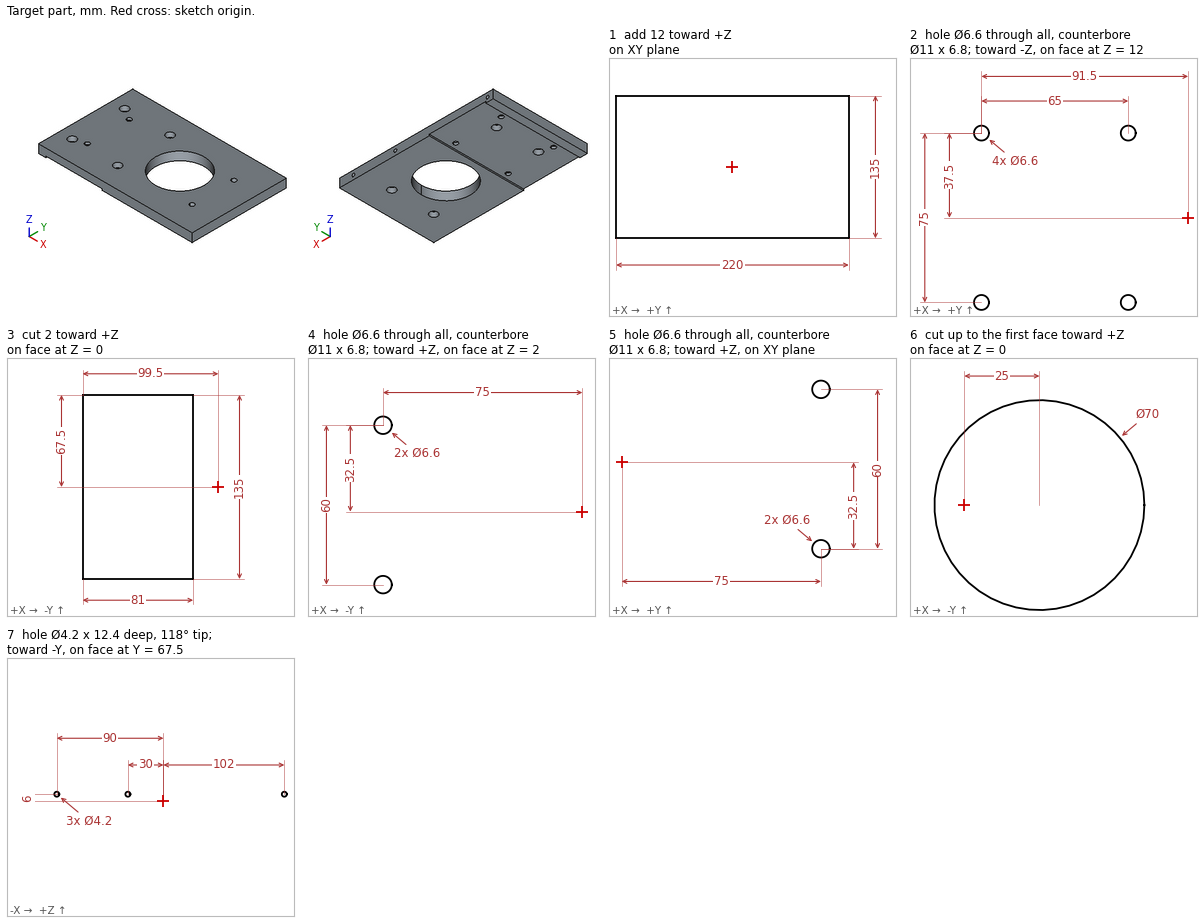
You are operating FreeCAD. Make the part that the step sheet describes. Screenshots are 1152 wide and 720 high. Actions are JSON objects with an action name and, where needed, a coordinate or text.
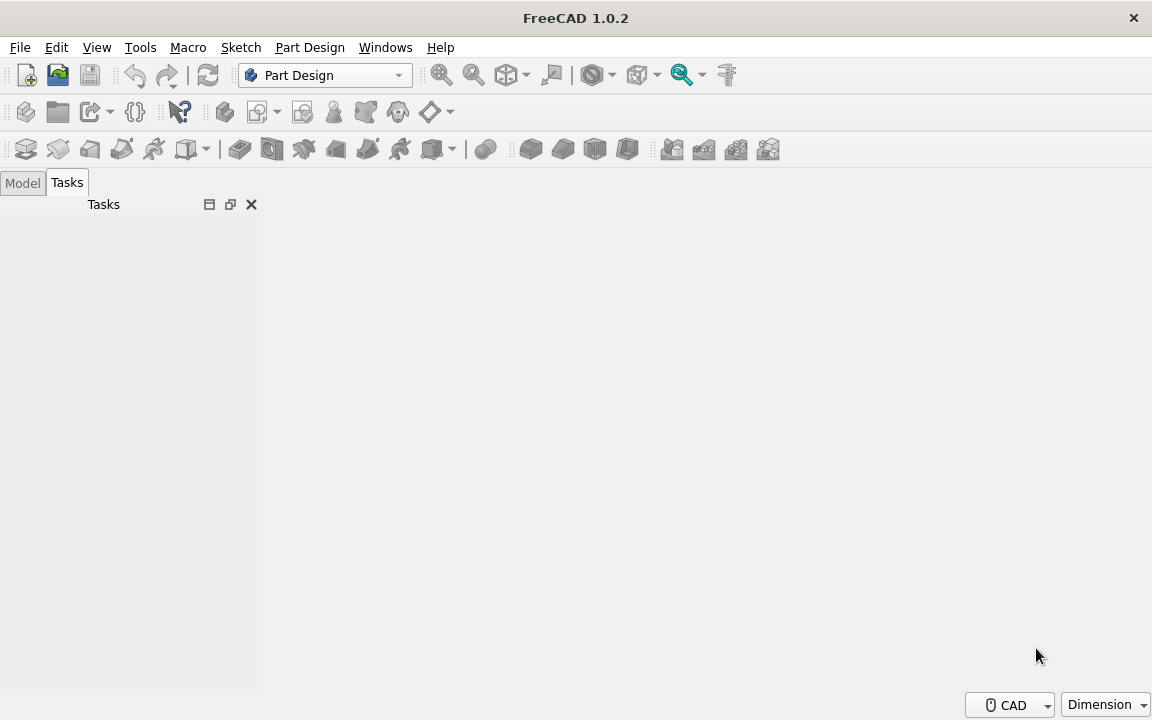
{"action": "key", "text": "ctrl+n"}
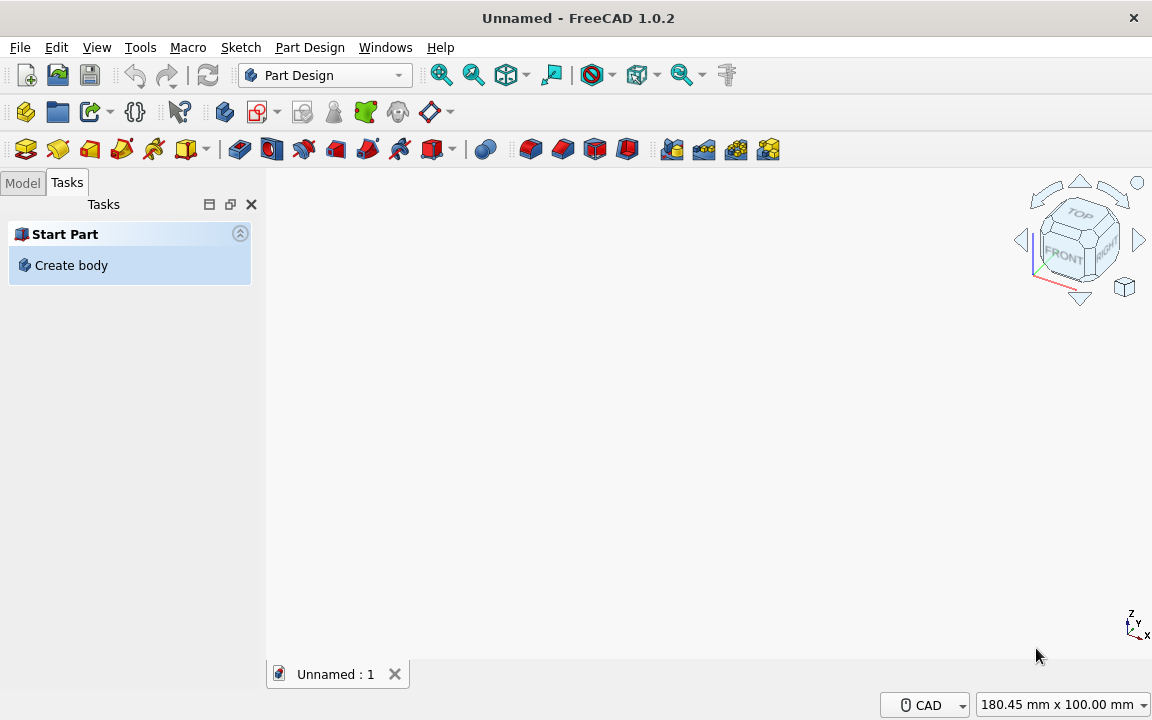
{"action": "left_click", "coordinate": [258, 112]}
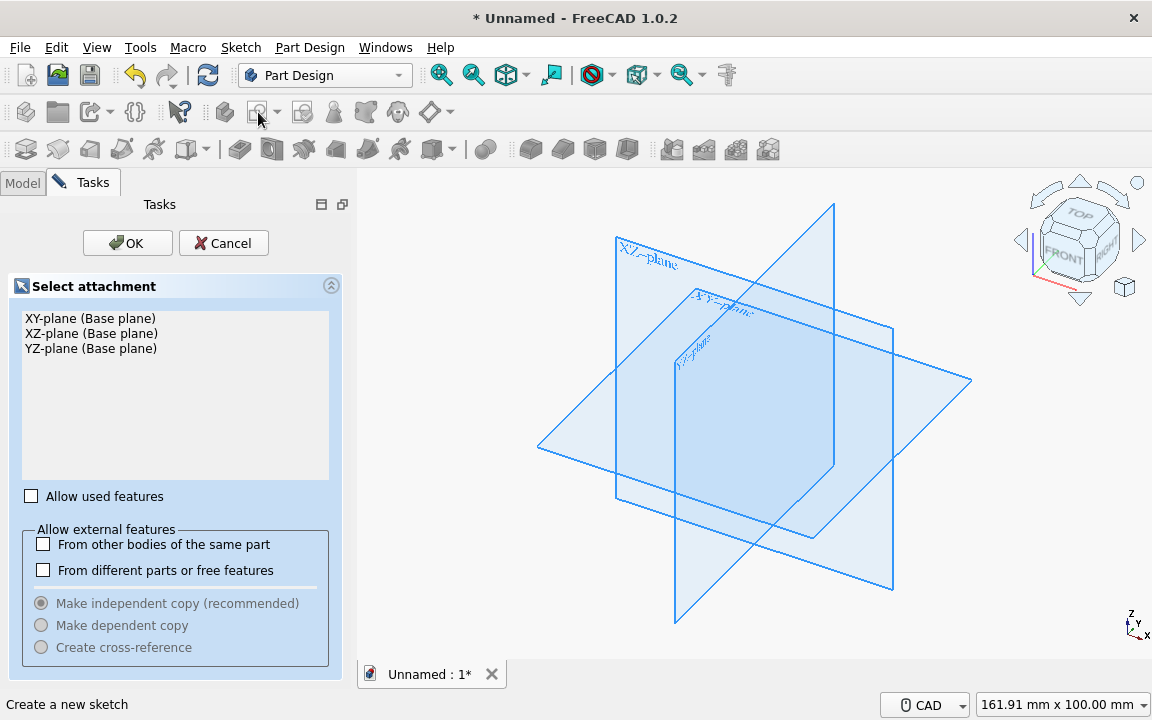
{"action": "left_click", "coordinate": [82, 318]}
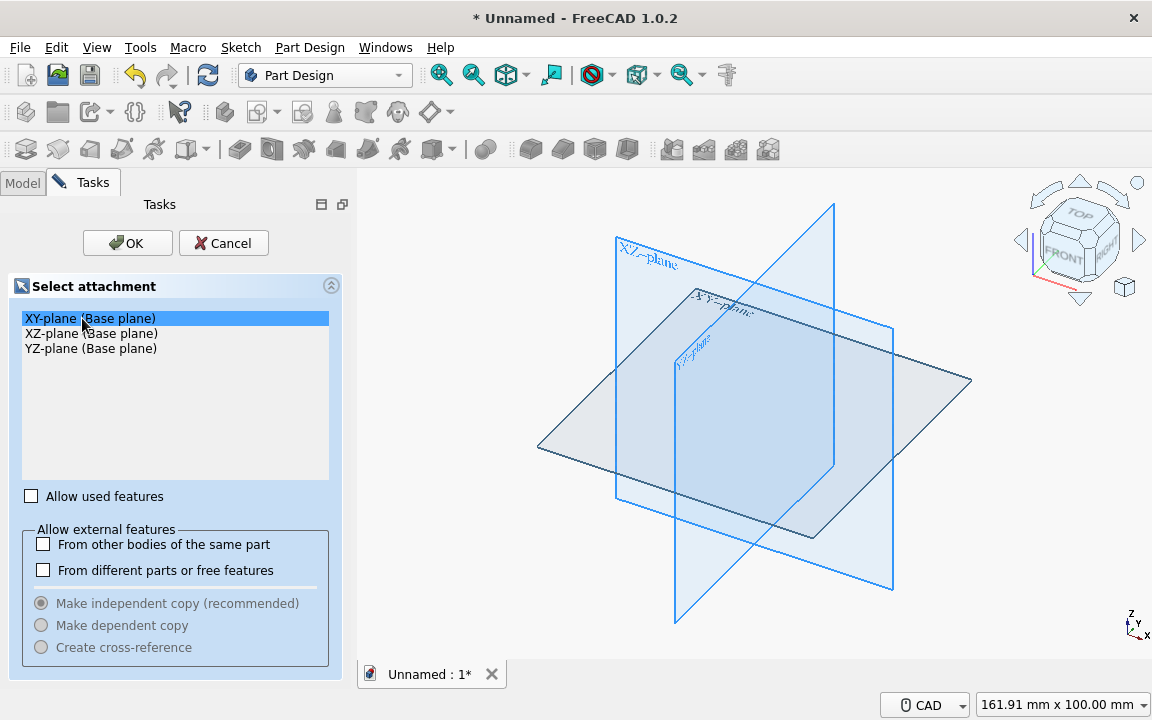
{"action": "left_click", "coordinate": [128, 243]}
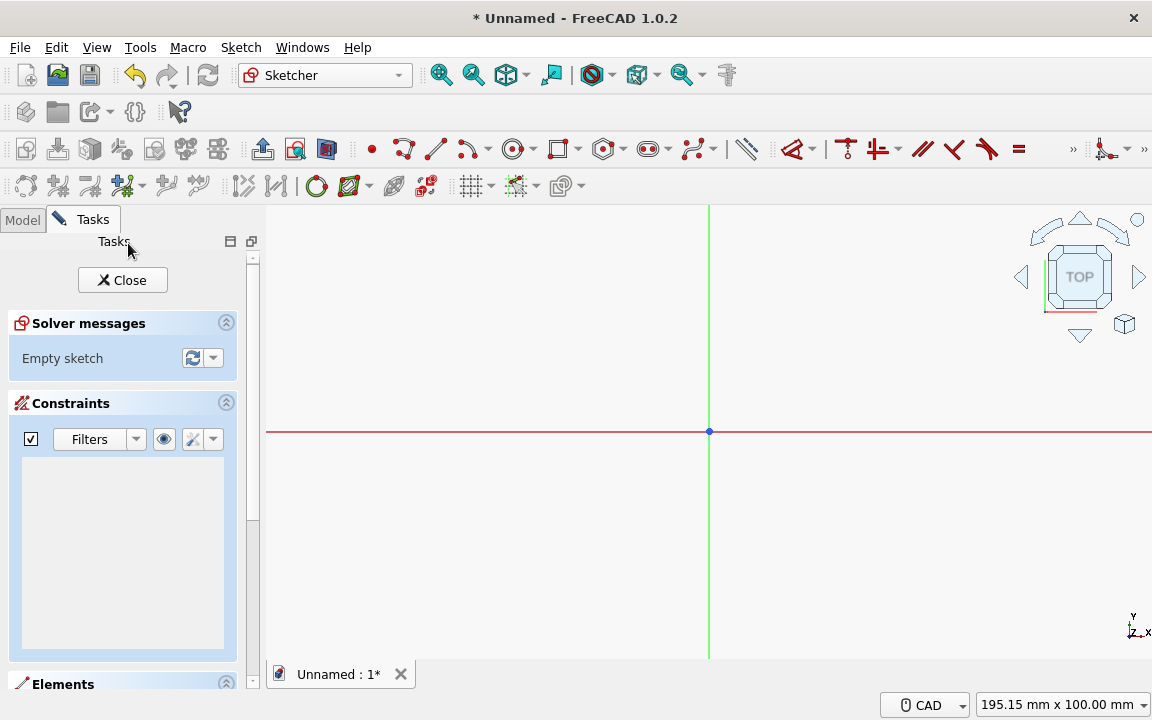
{"action": "scroll", "coordinate": [585, 432], "scroll_direction": "down", "scroll_amount": 4}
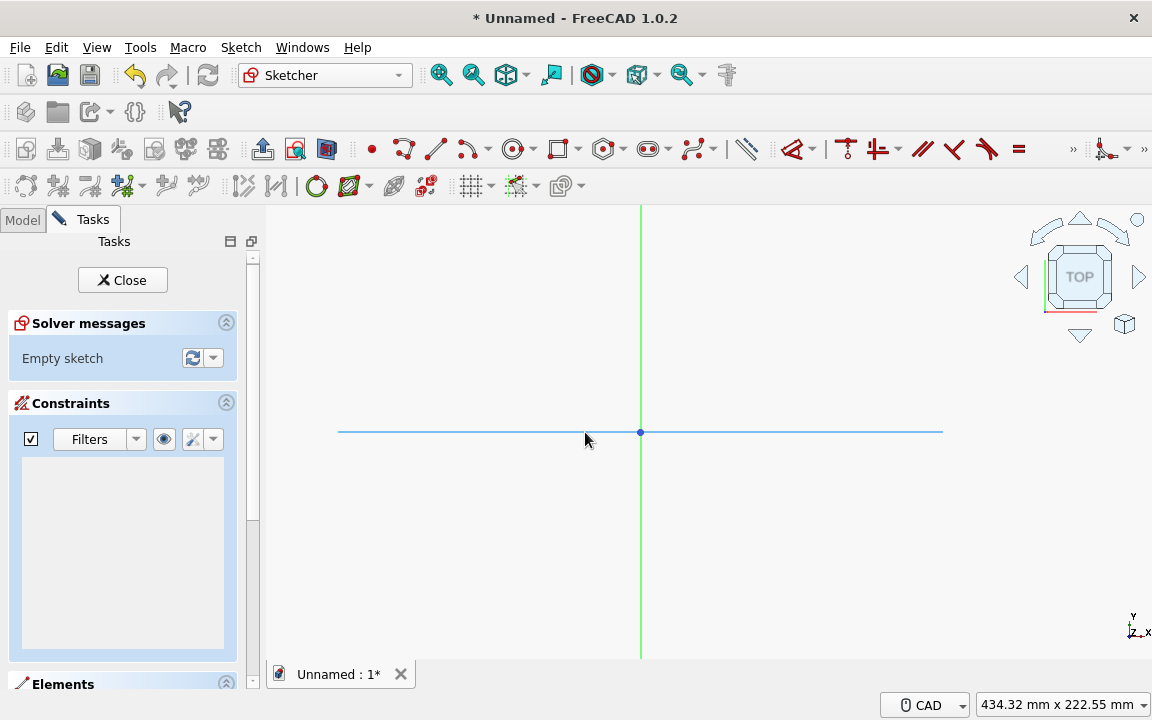
{"action": "left_click", "coordinate": [580, 150]}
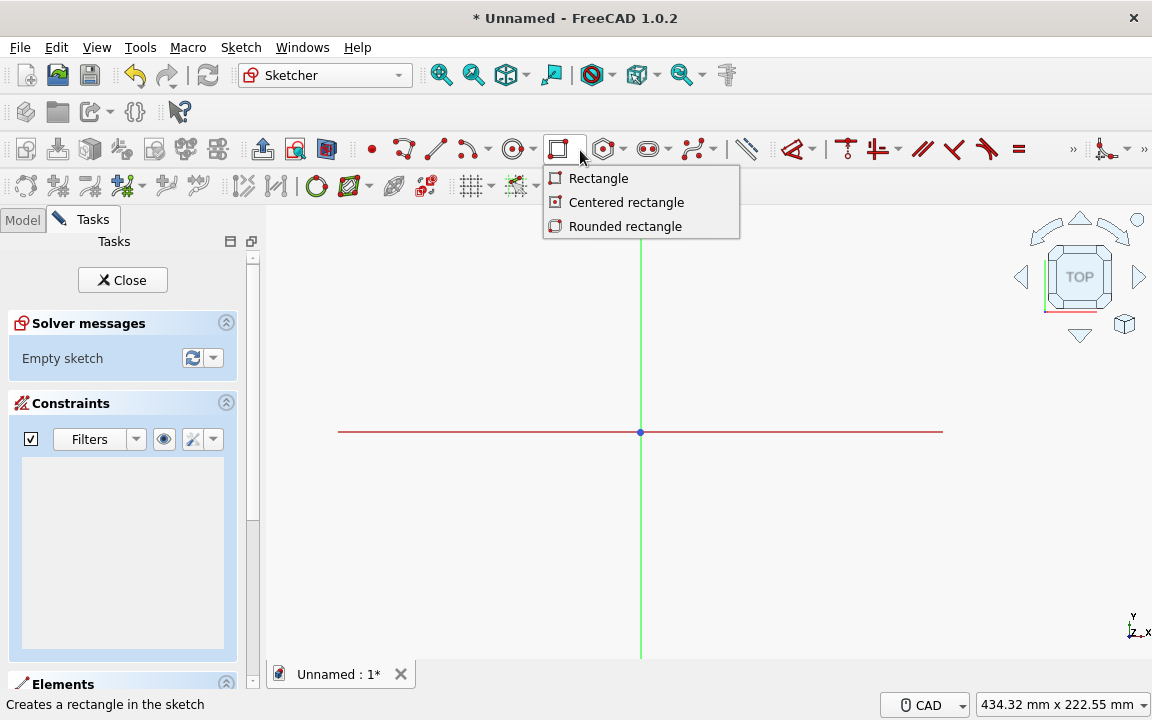
{"action": "left_click", "coordinate": [642, 202]}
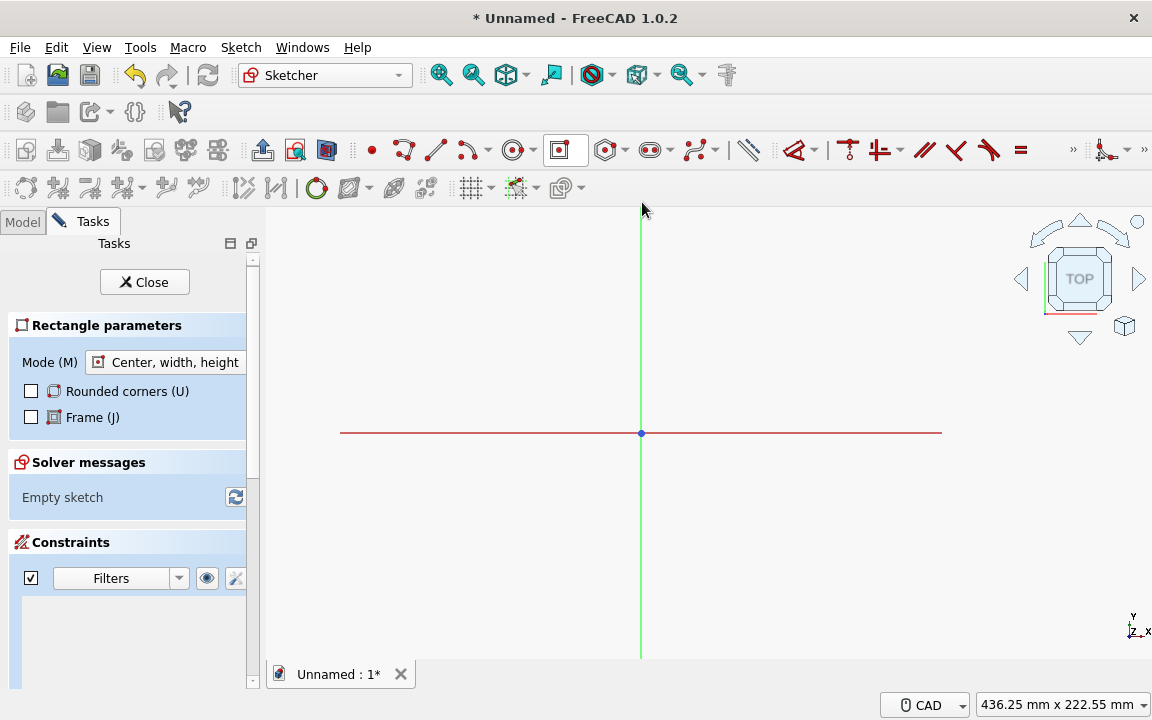
{"action": "left_click", "coordinate": [641, 433]}
{"action": "mouse_move", "coordinate": [865, 296]}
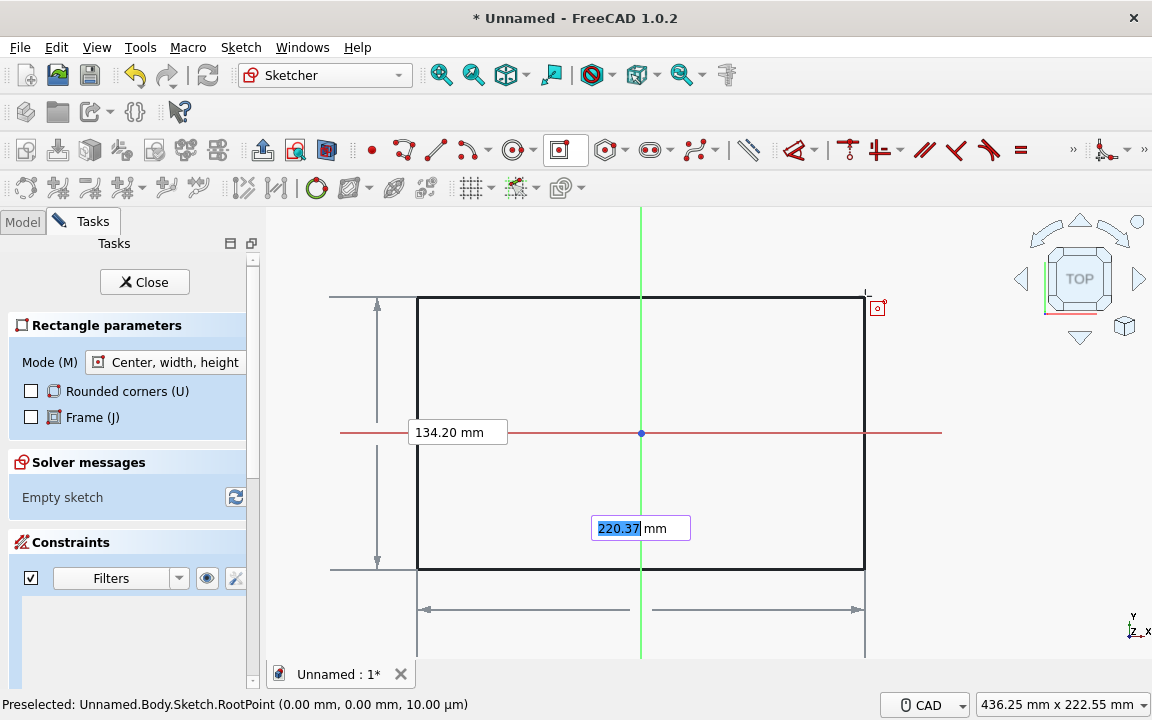
{"action": "type", "text": "220"}
{"action": "key", "text": "Tab"}
{"action": "type", "text": "135"}
{"action": "key", "text": "Return"}
{"action": "key", "text": "Escape"}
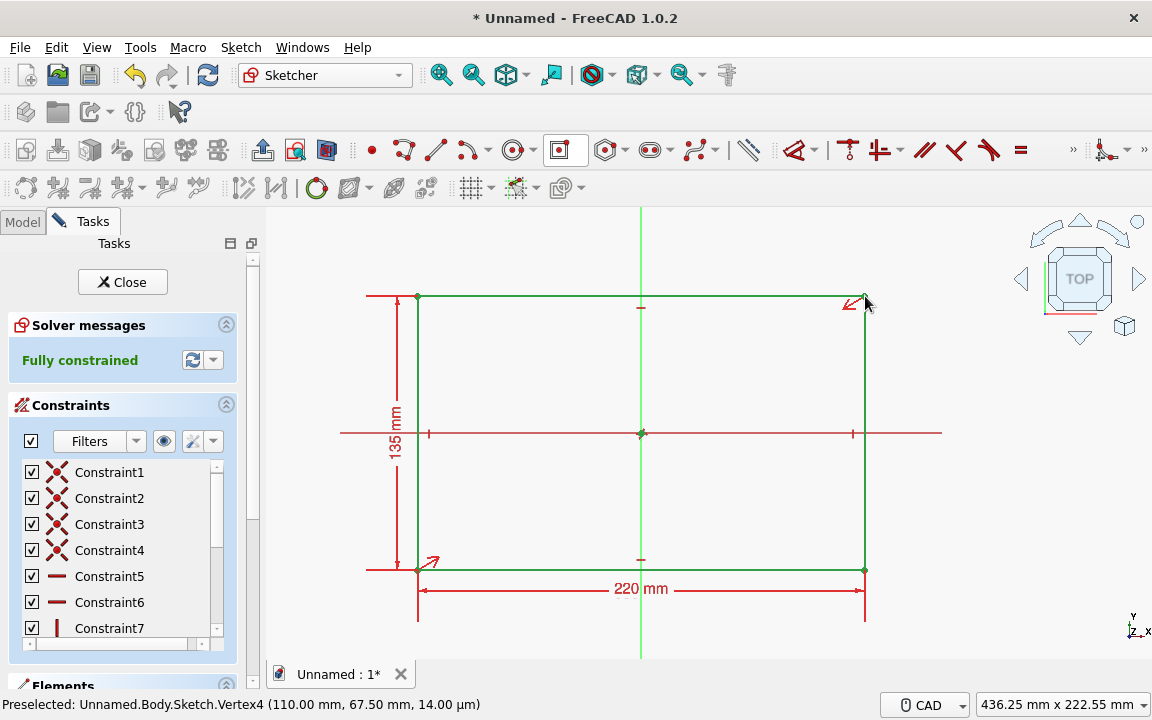
{"action": "left_click", "coordinate": [123, 282]}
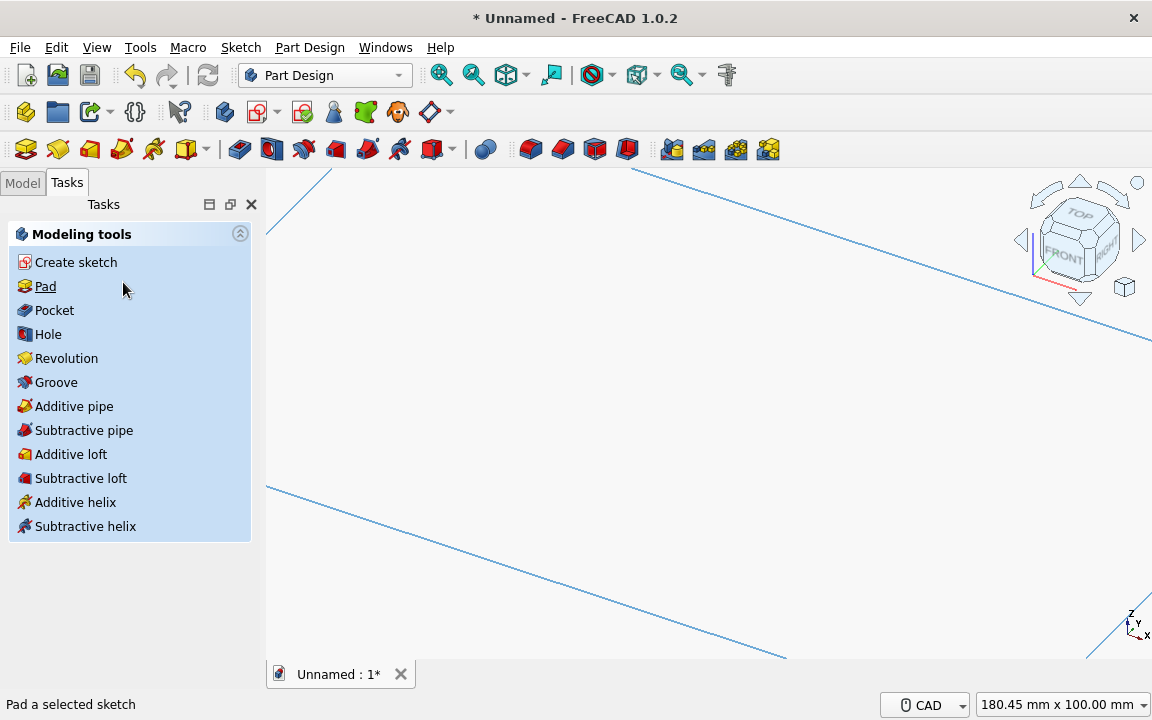
{"action": "left_click", "coordinate": [26, 150]}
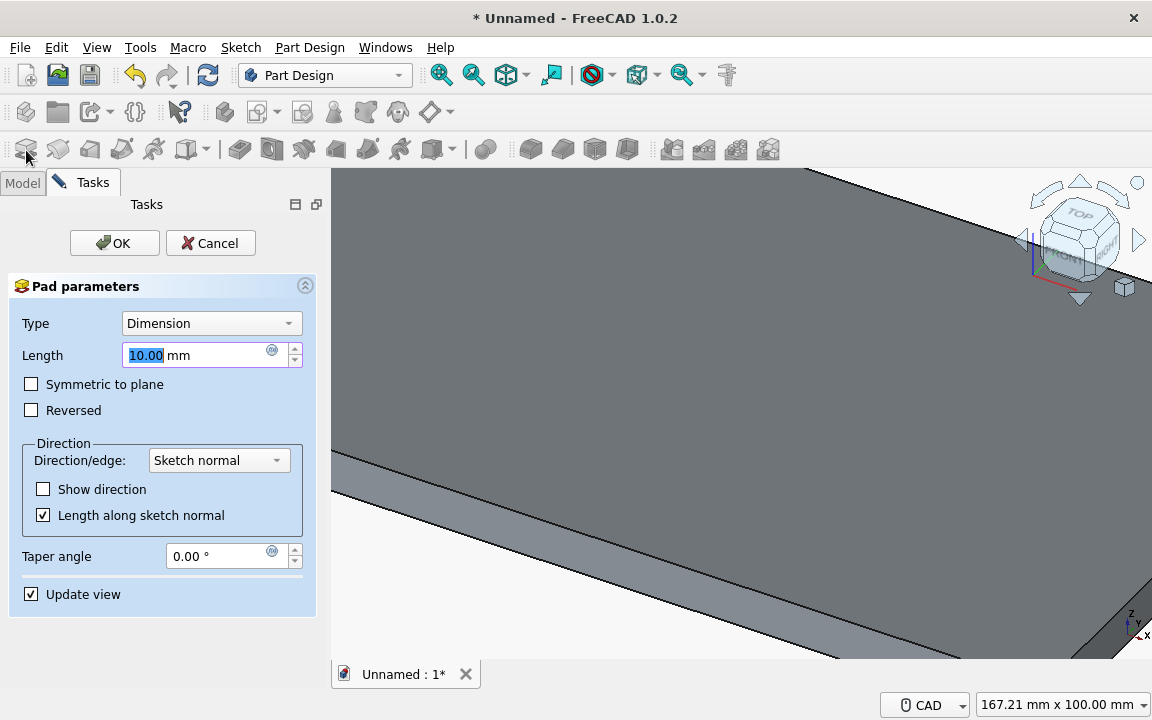
{"action": "type", "text": "12"}
{"action": "key", "text": "Tab"}